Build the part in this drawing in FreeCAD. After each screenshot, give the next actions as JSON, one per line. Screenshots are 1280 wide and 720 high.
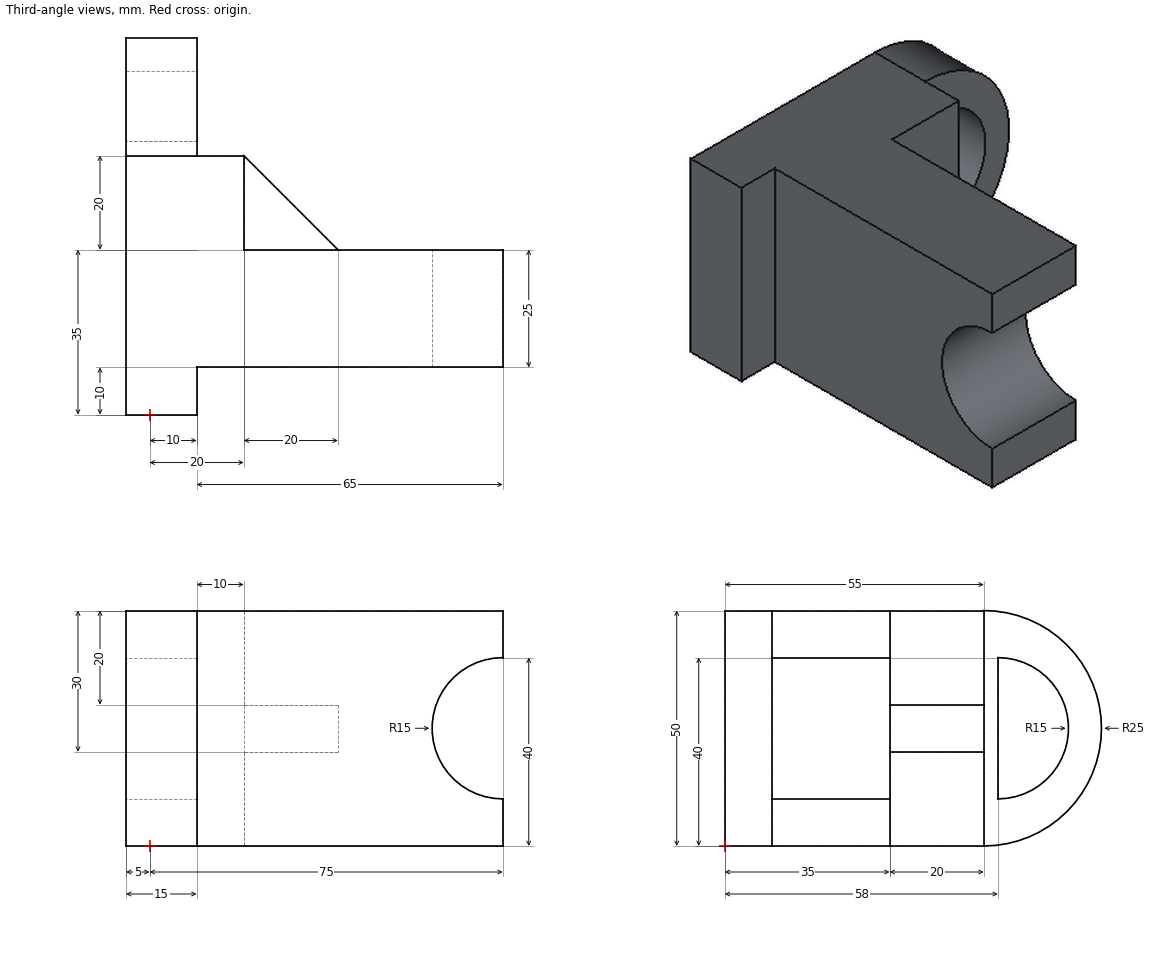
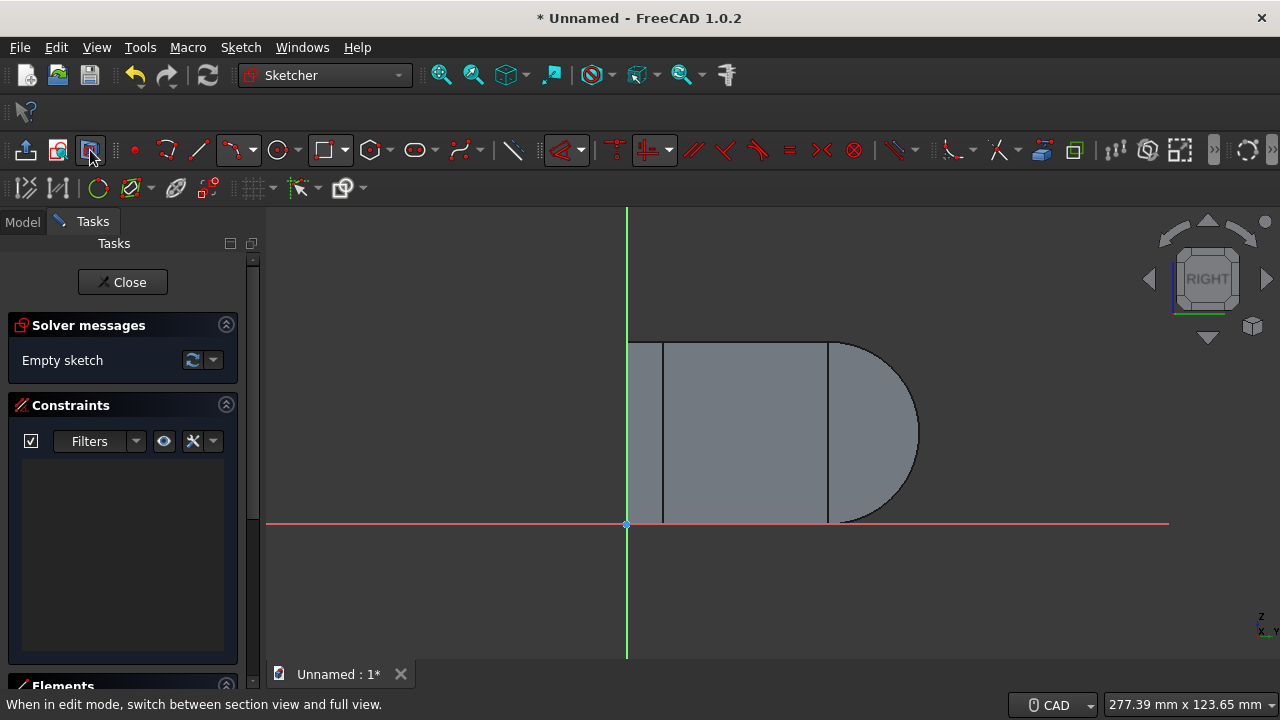
{"action": "scroll", "coordinate": [828, 474], "scroll_direction": "up", "scroll_amount": 3}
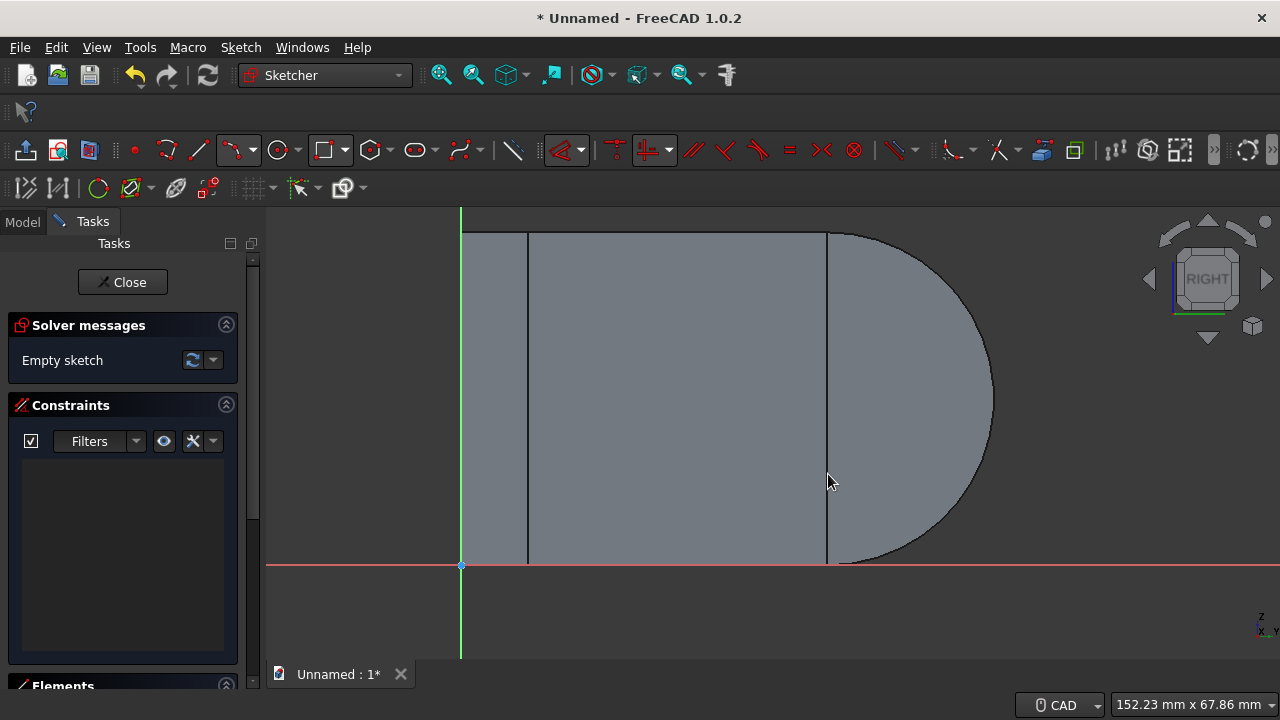
{"action": "key", "text": "g l"}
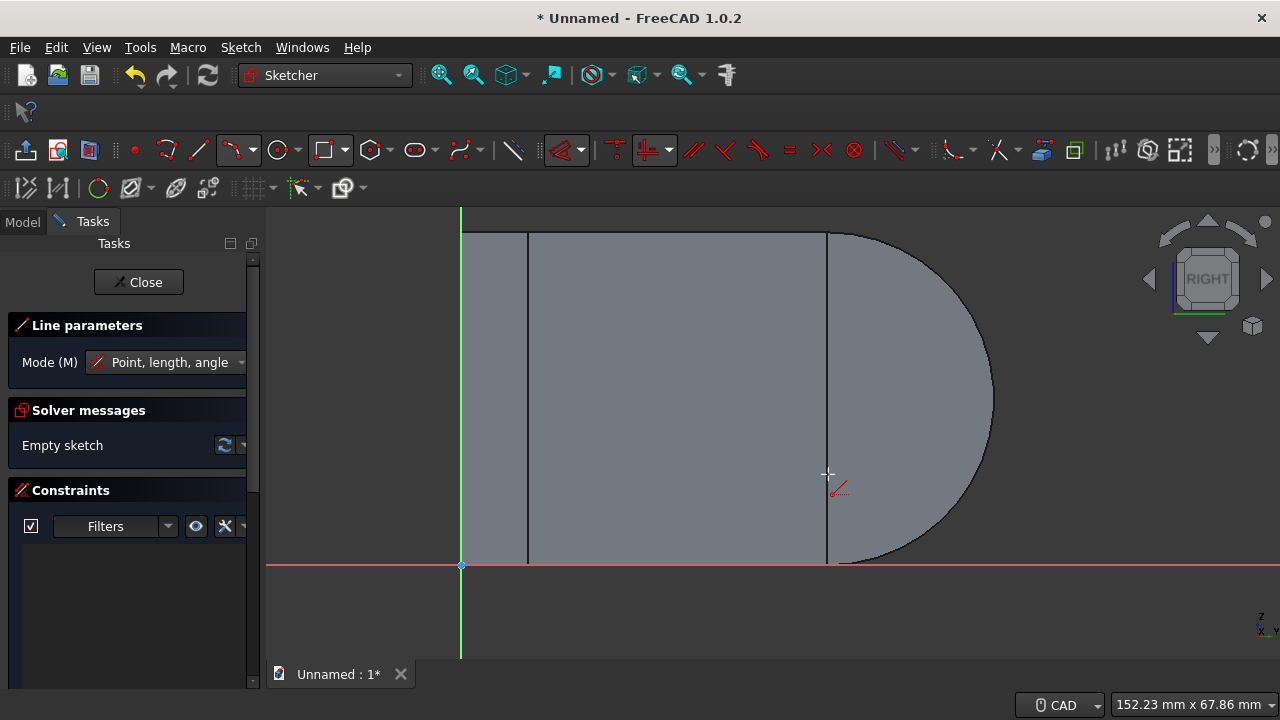
{"action": "left_click", "coordinate": [847, 299]}
{"action": "left_click", "coordinate": [847, 499]}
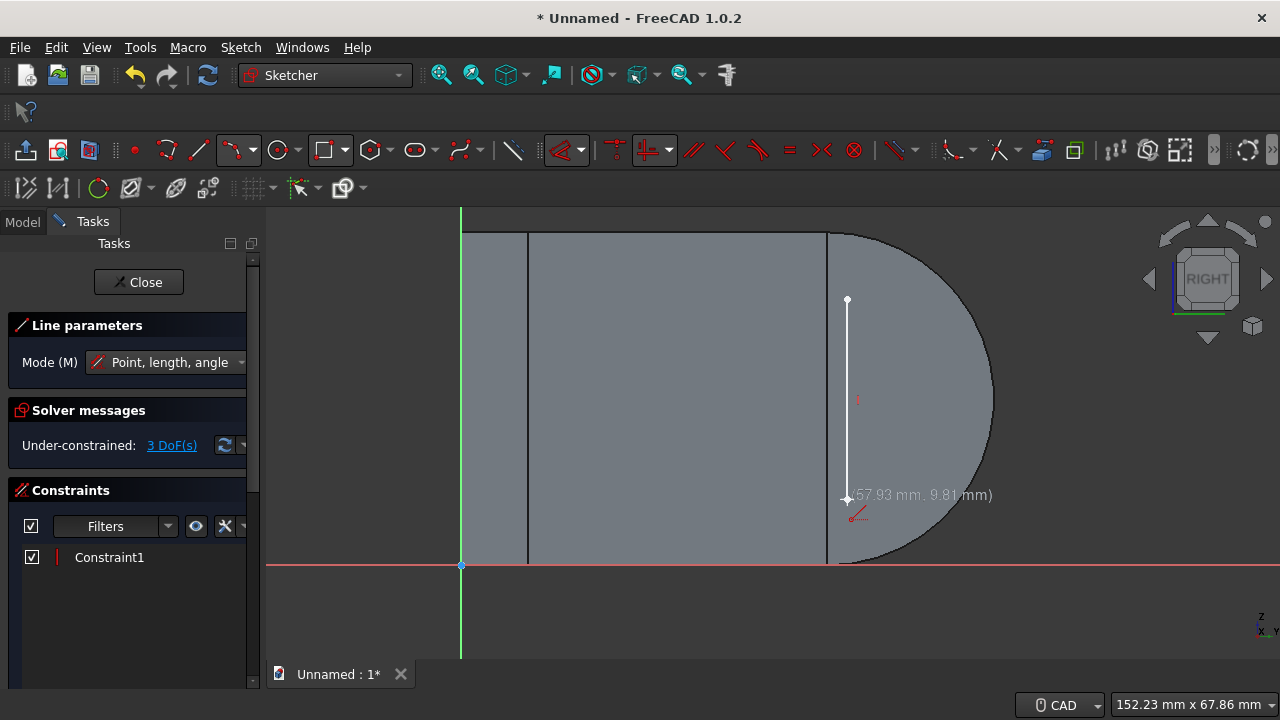
{"action": "left_click", "coordinate": [232, 150]}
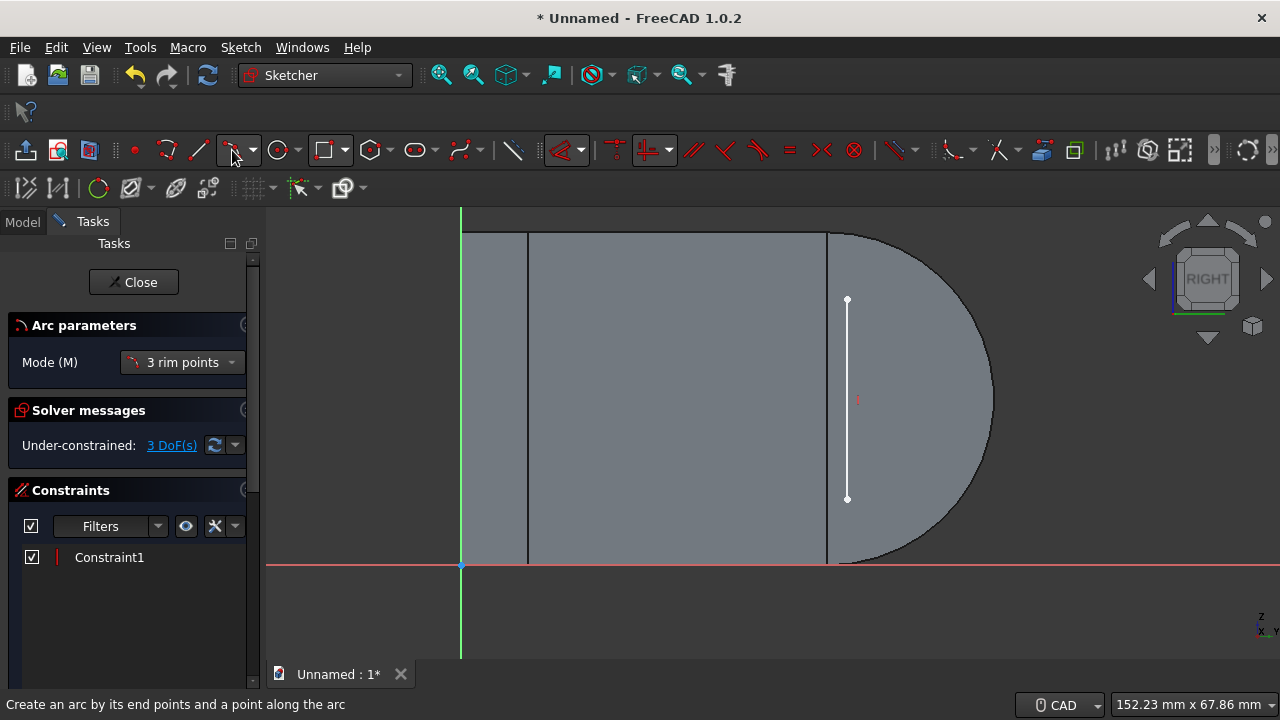
{"action": "left_click", "coordinate": [847, 500]}
{"action": "left_click", "coordinate": [847, 300]}
{"action": "left_click", "coordinate": [947, 399]}
{"action": "key", "text": "Escape"}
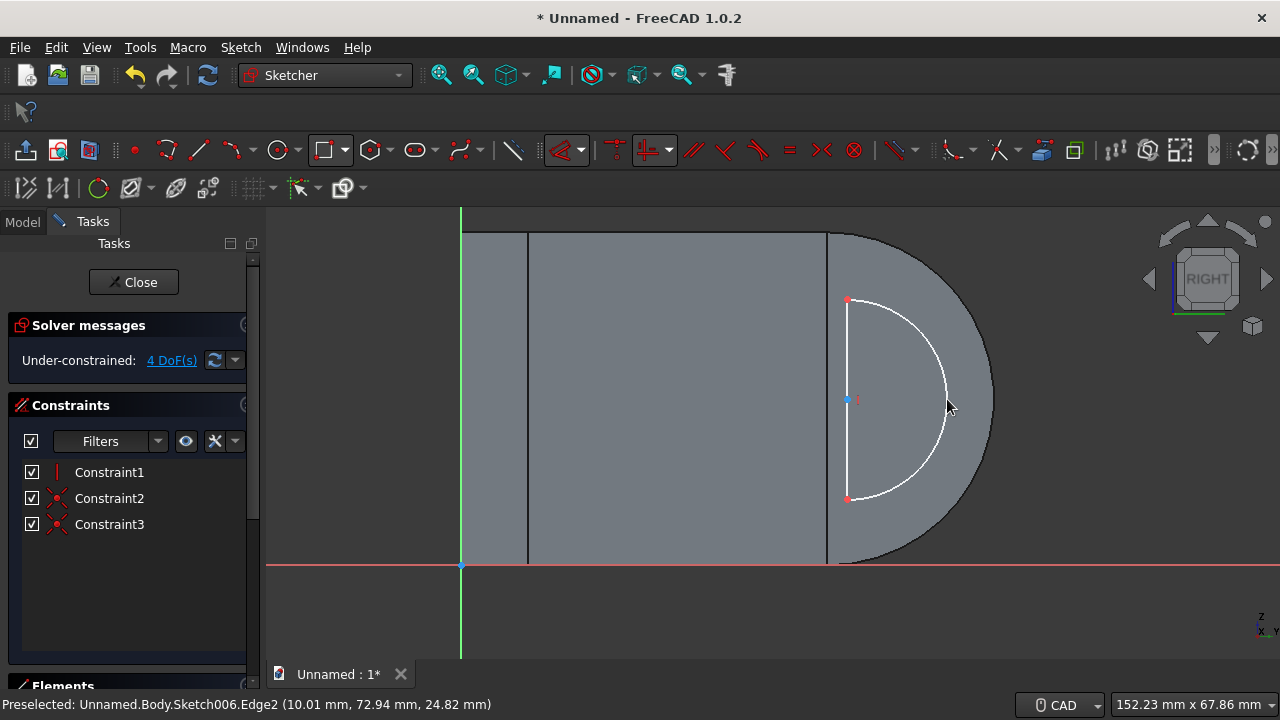
{"action": "left_click", "coordinate": [928, 459]}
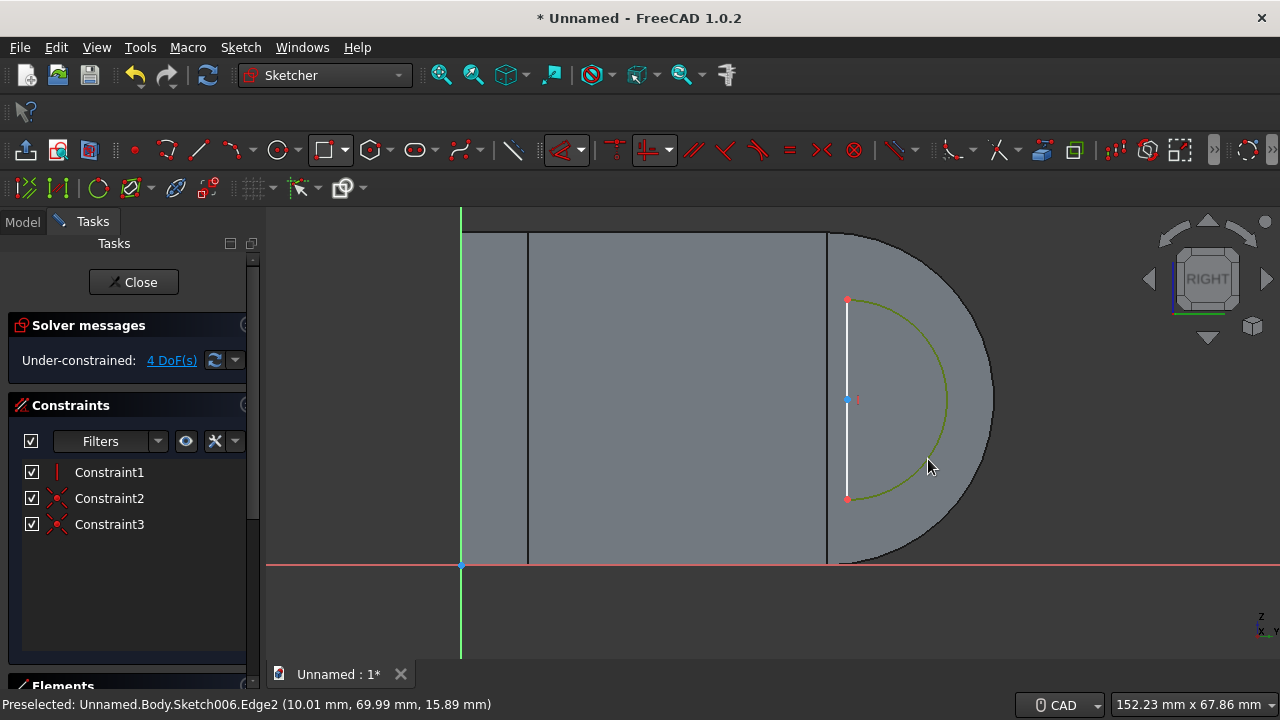
{"action": "left_click", "coordinate": [584, 150]}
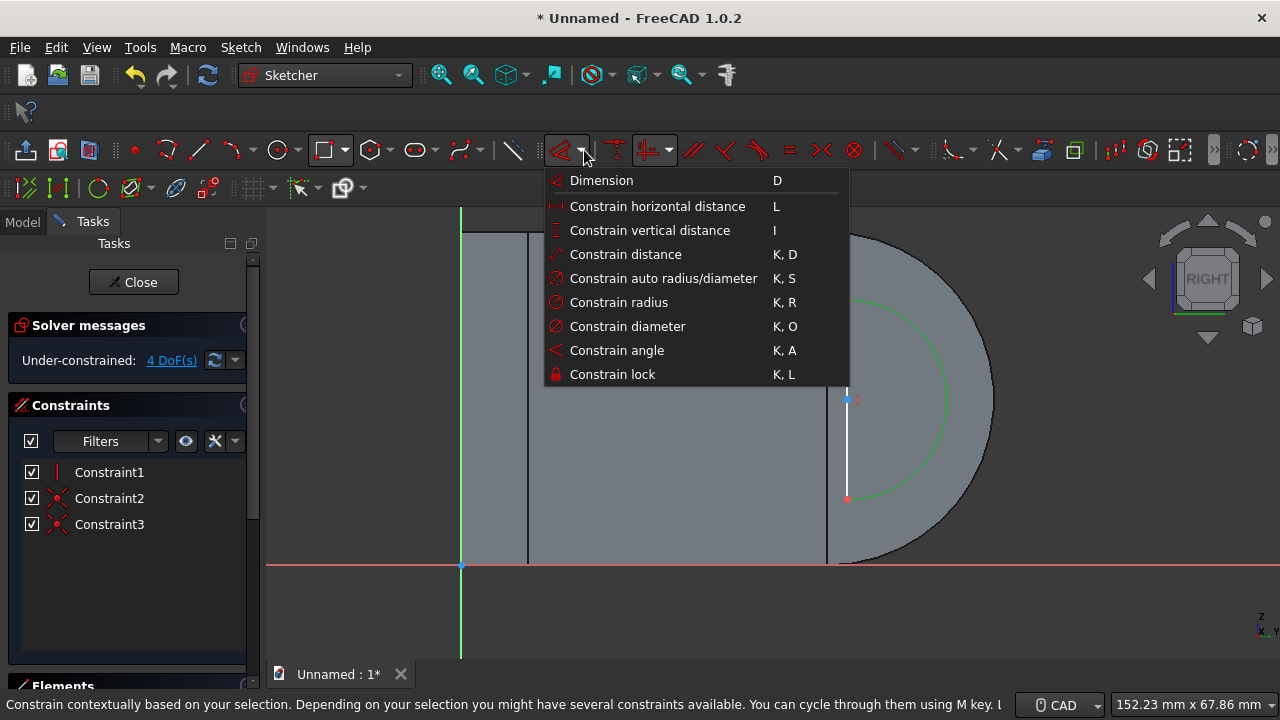
{"action": "left_click", "coordinate": [697, 302]}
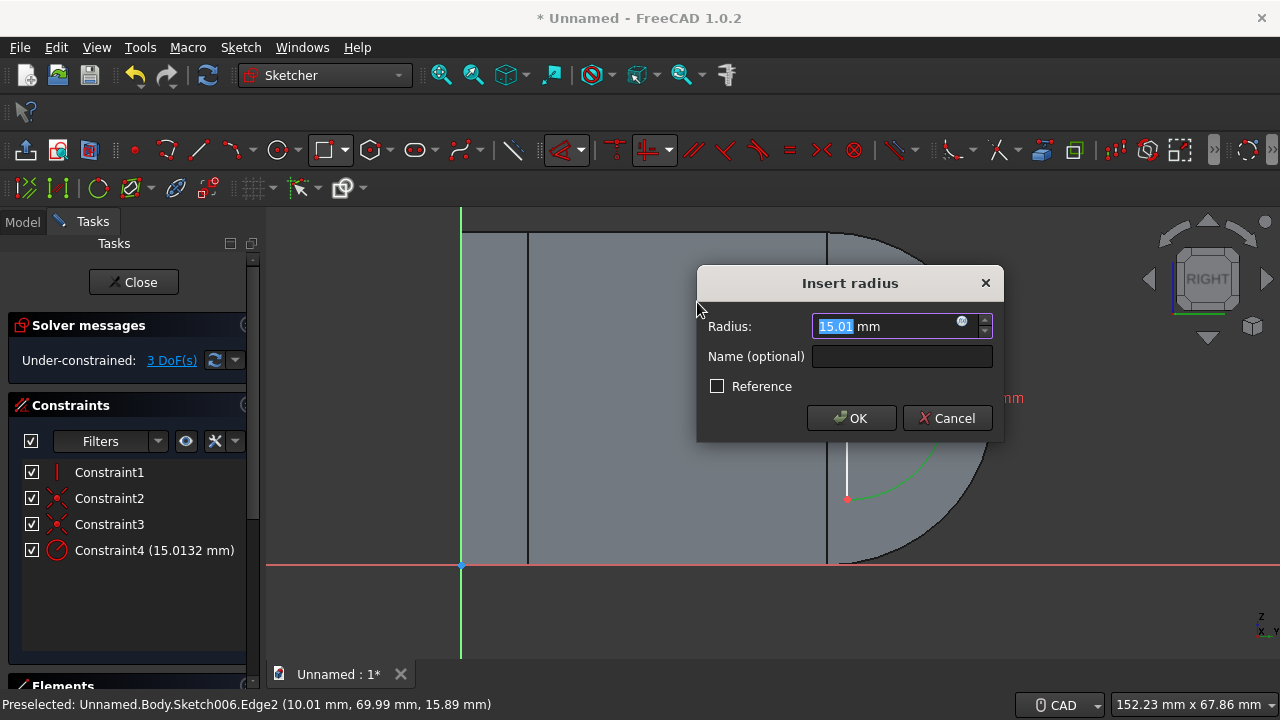
{"action": "type", "text": "15"}
{"action": "key", "text": "Return"}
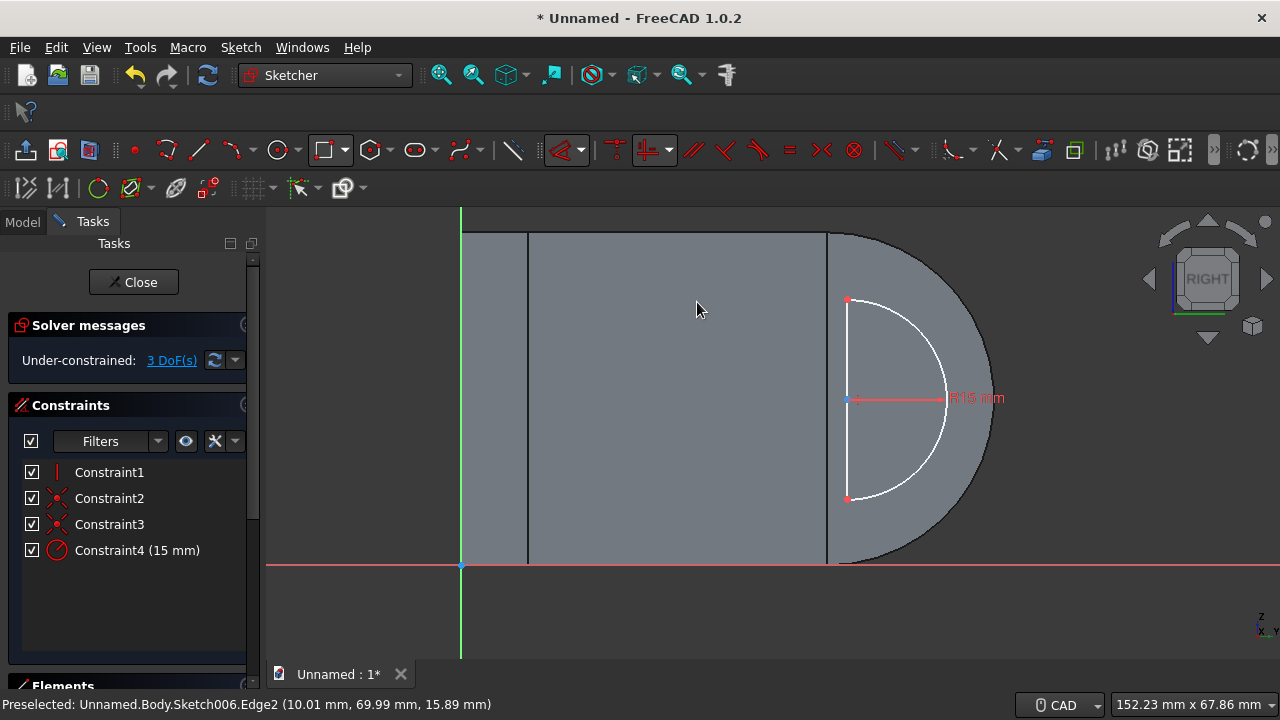
{"action": "left_click", "coordinate": [847, 300]}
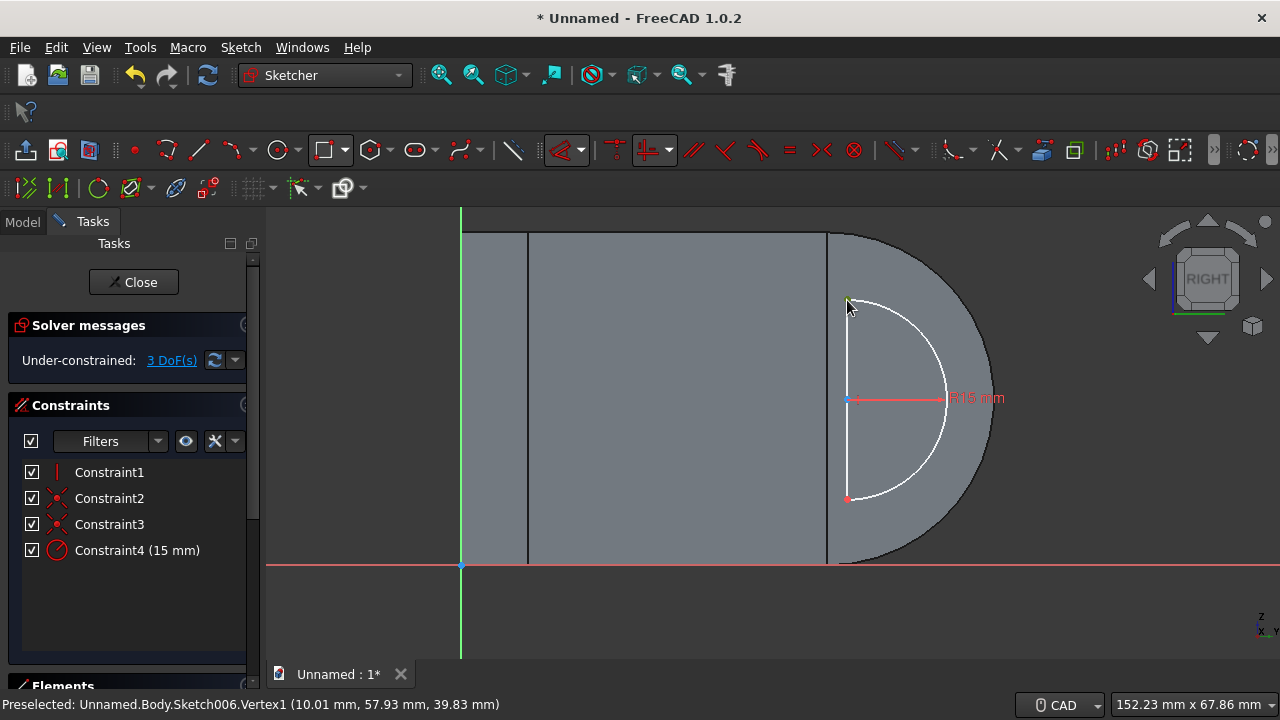
{"action": "left_click", "coordinate": [584, 150]}